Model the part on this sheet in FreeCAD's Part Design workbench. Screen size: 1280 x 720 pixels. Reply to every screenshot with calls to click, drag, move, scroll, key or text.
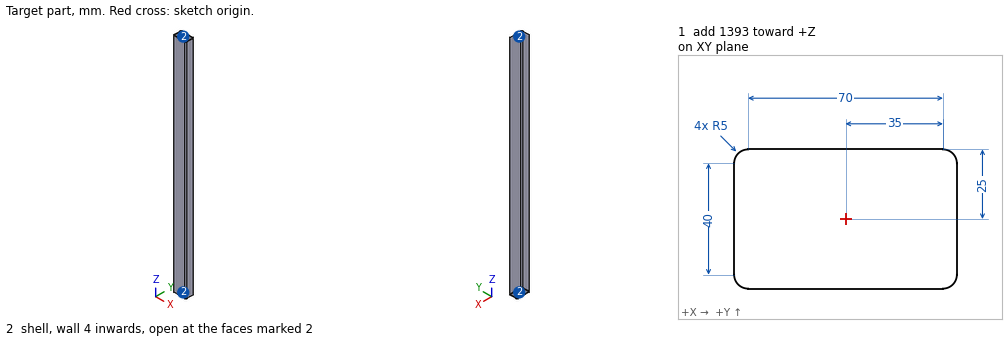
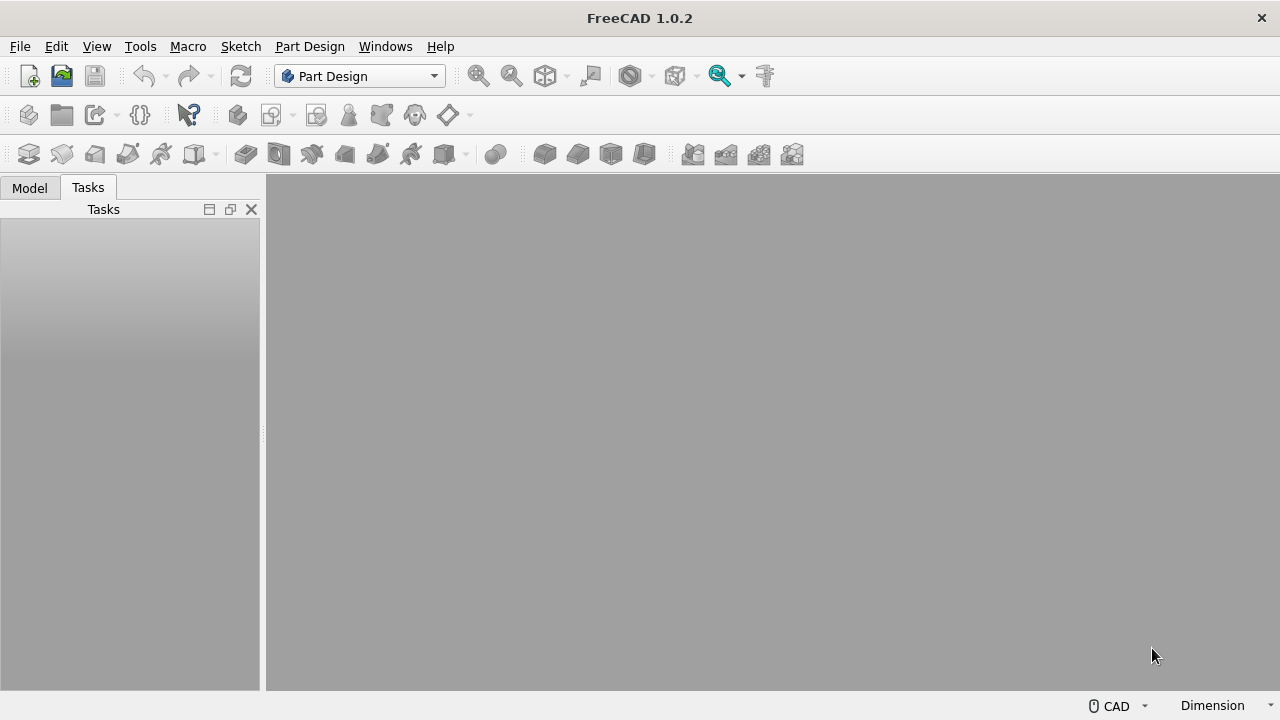
click(29, 76)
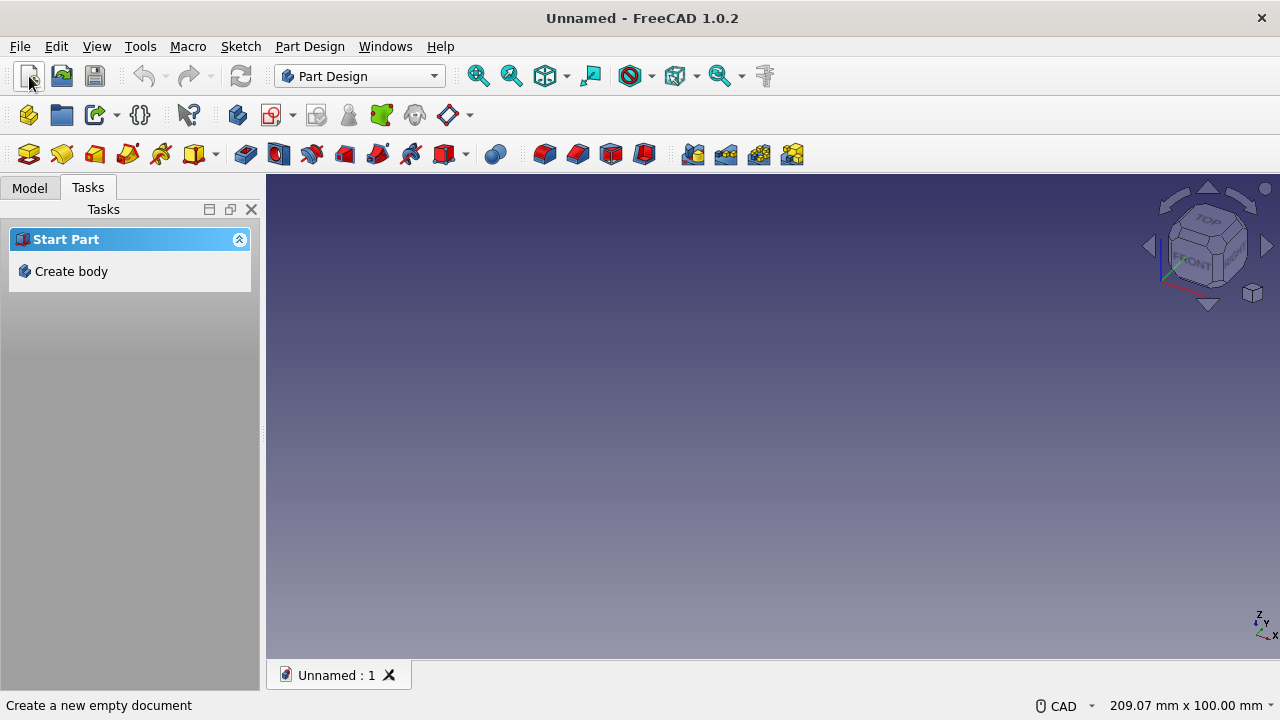
click(270, 116)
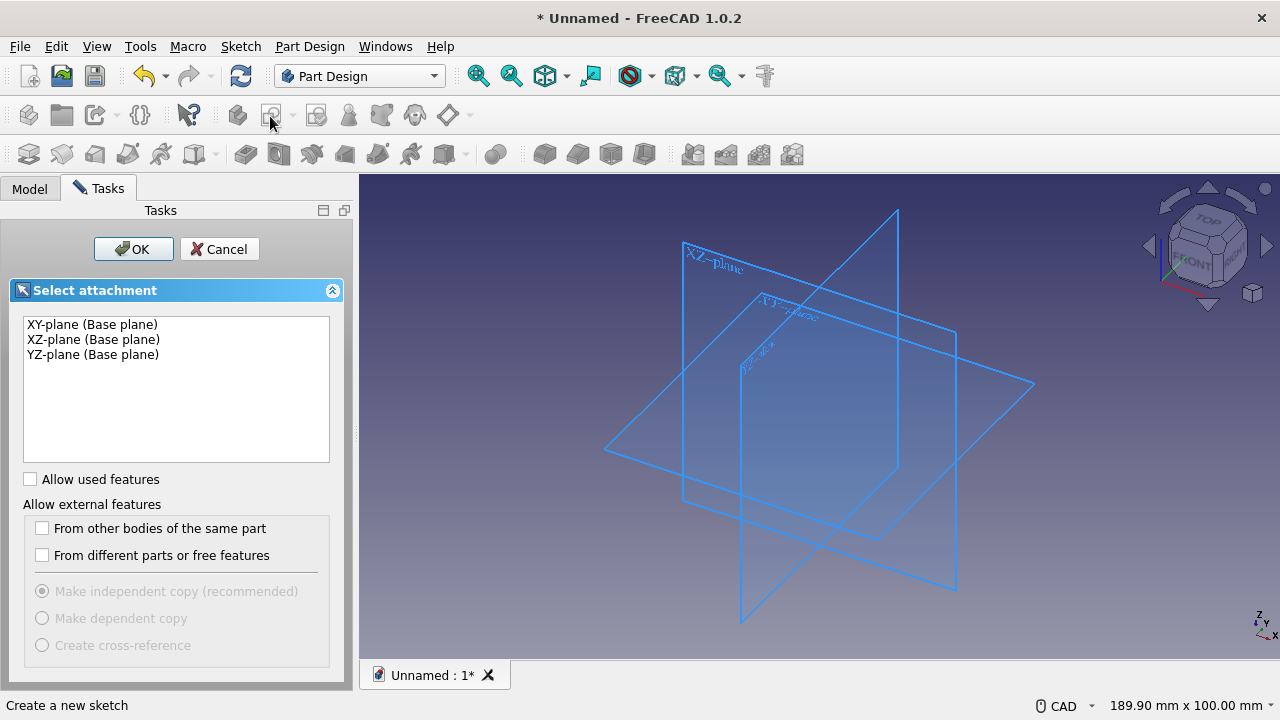
click(84, 324)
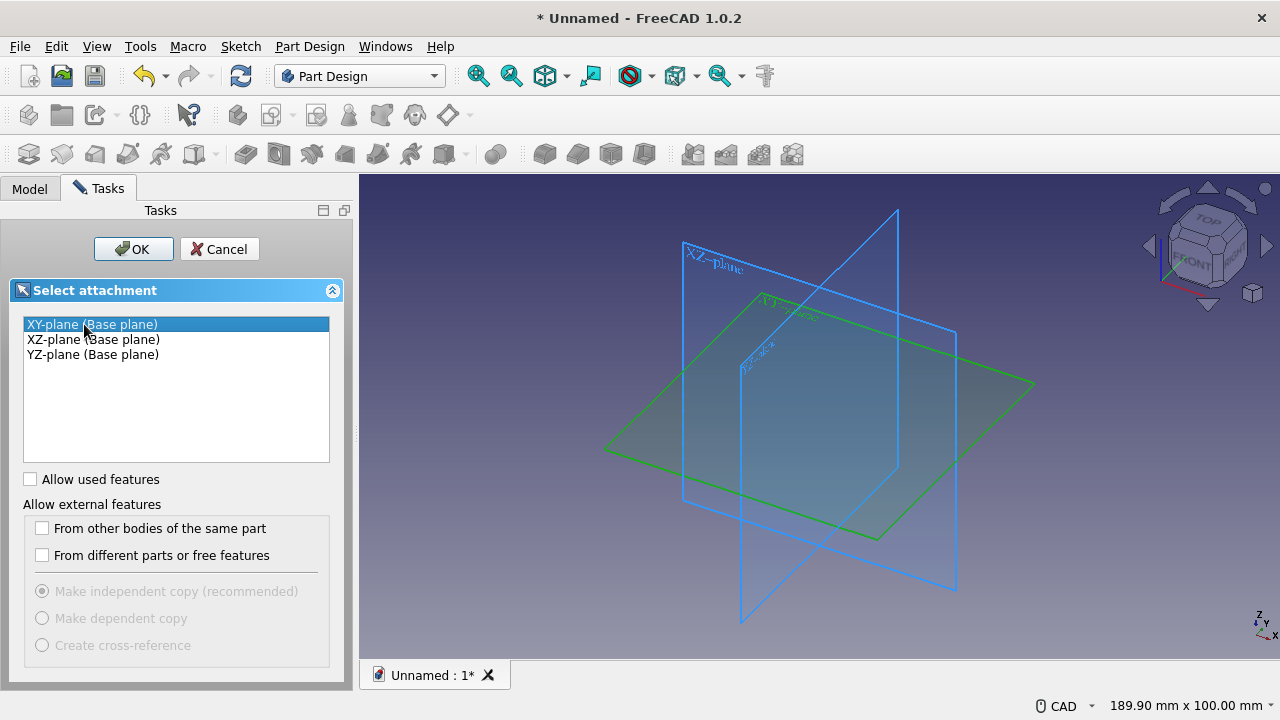
click(134, 249)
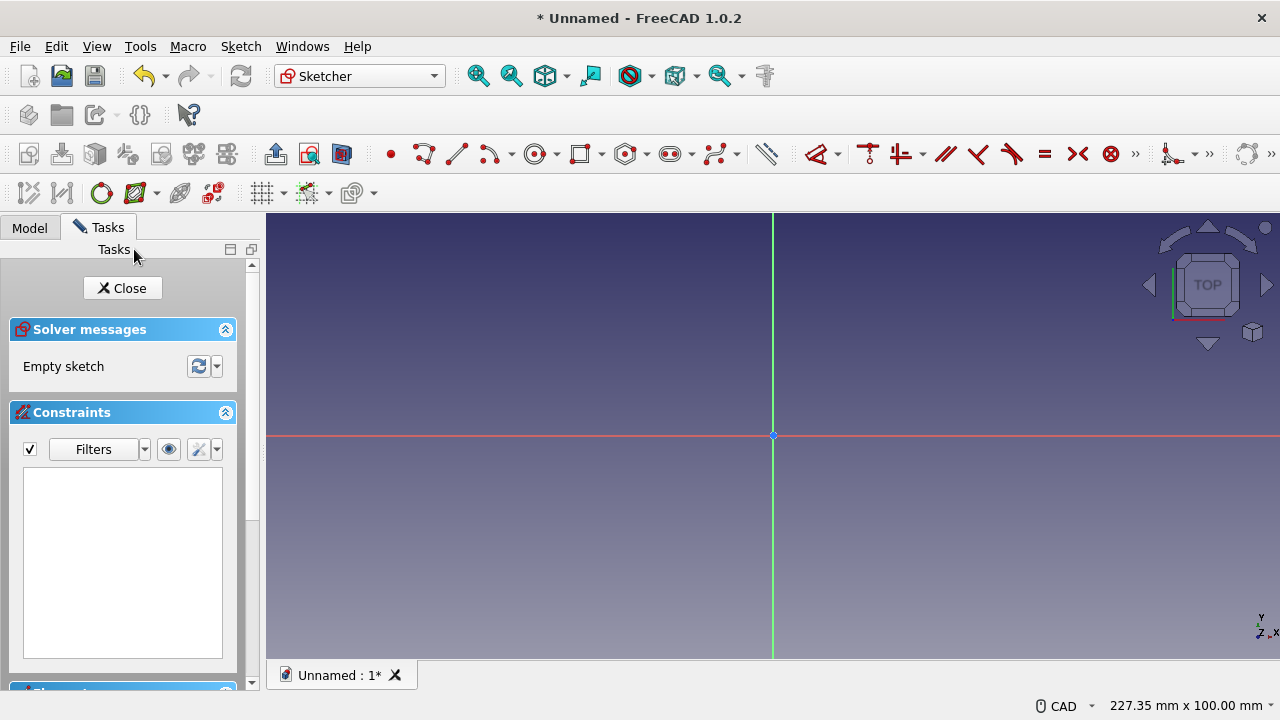
click(457, 154)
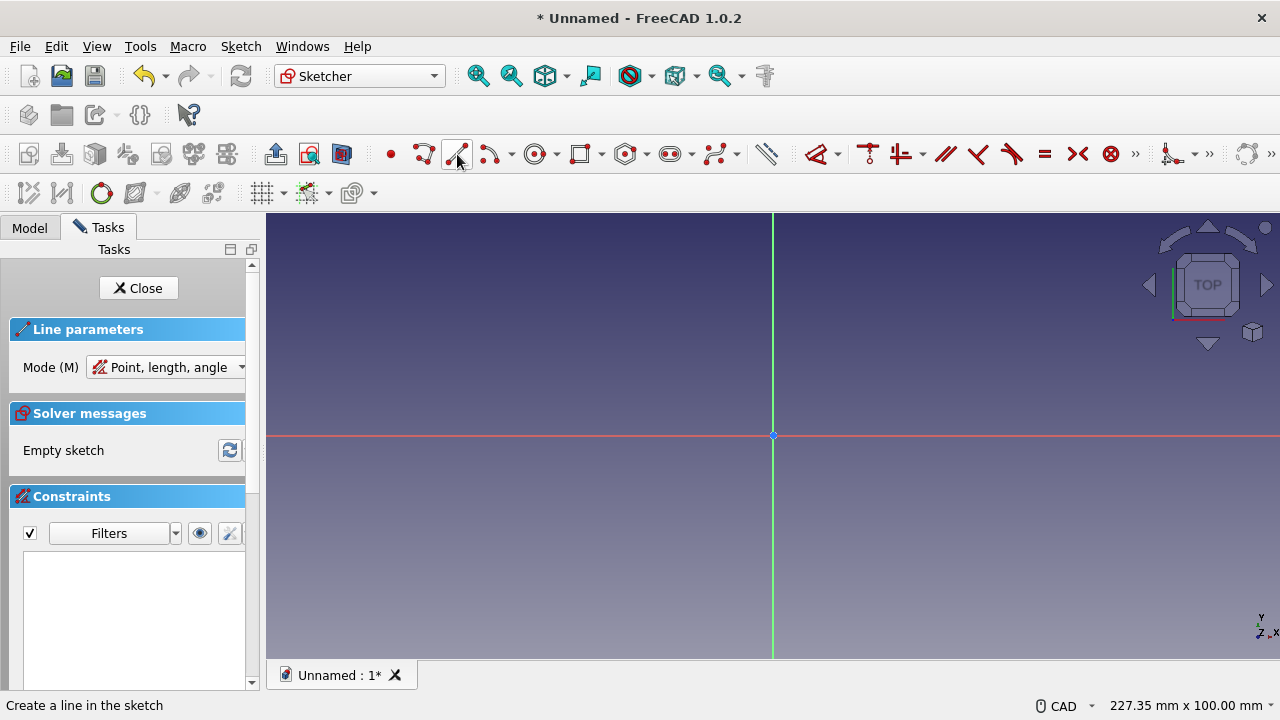
click(929, 324)
click(617, 324)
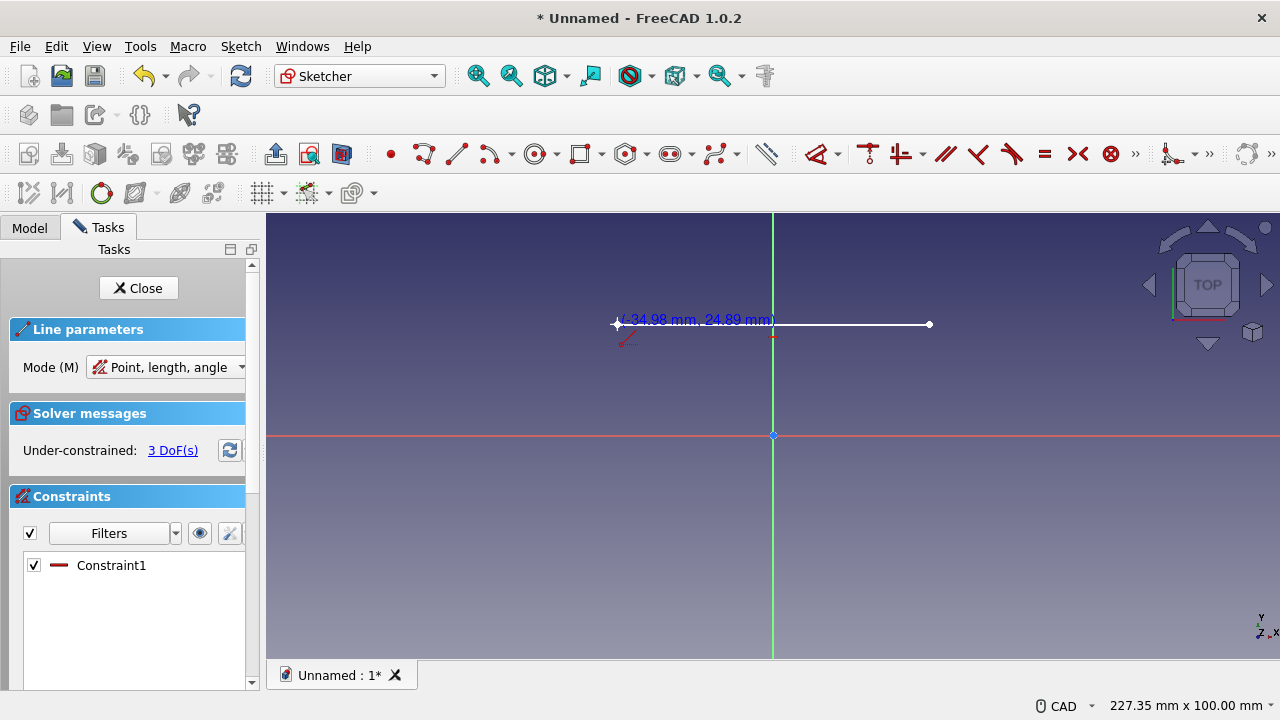
click(595, 347)
click(595, 525)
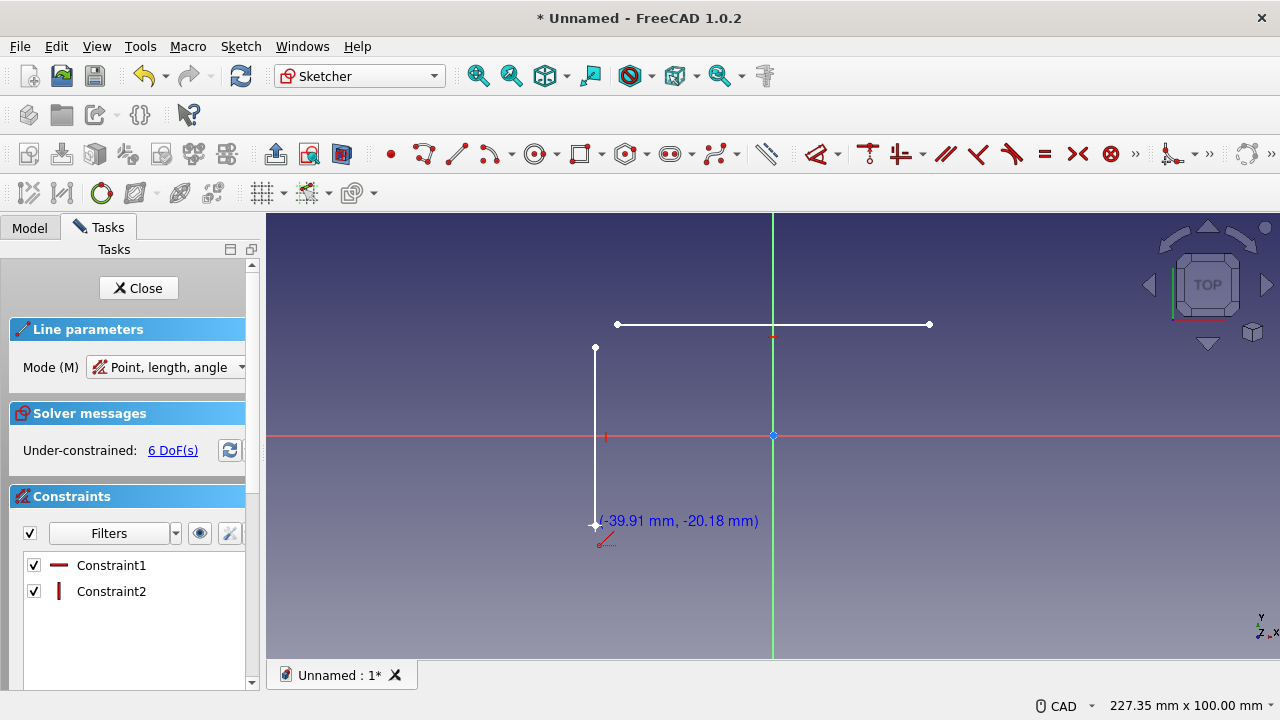
click(617, 548)
click(929, 548)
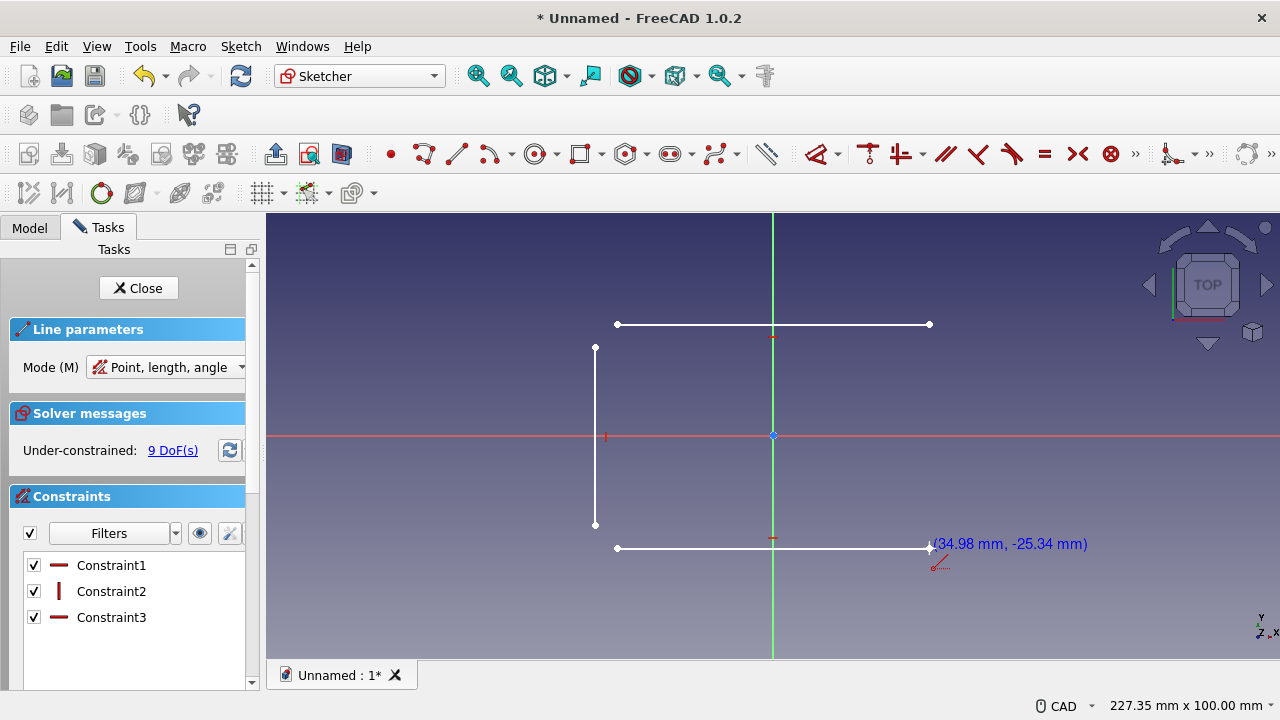
click(951, 525)
click(951, 347)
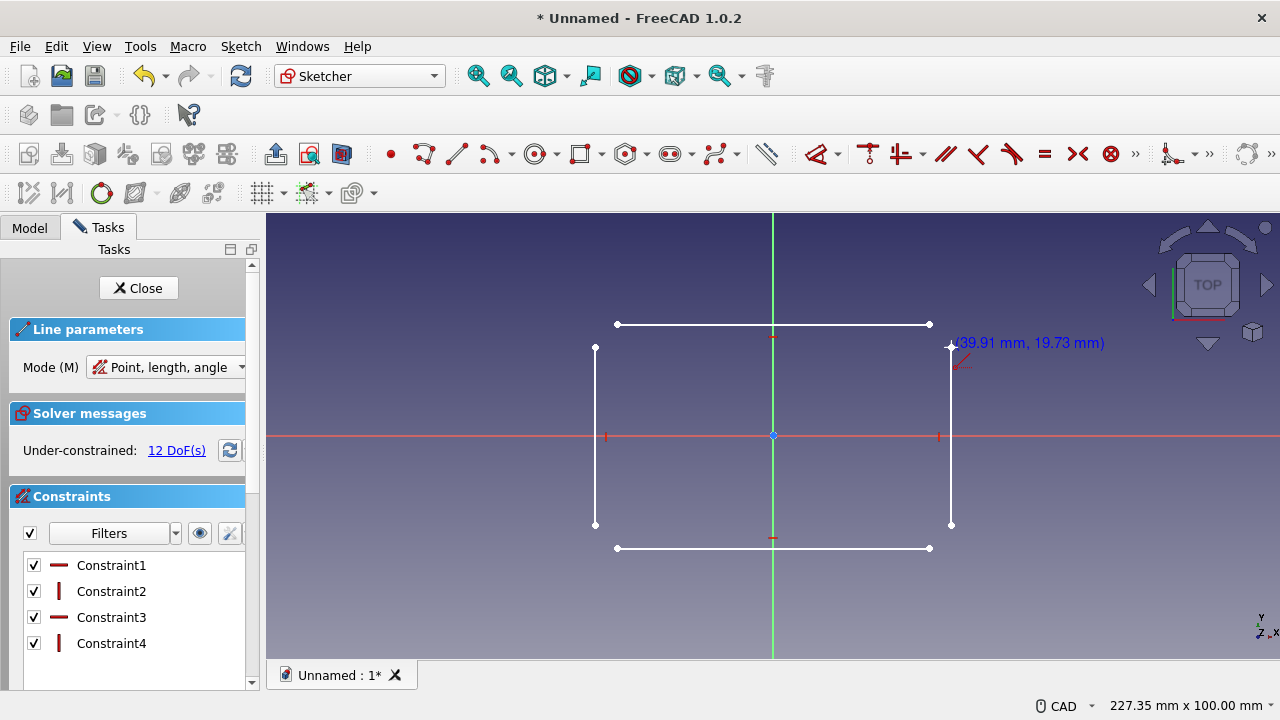
click(512, 154)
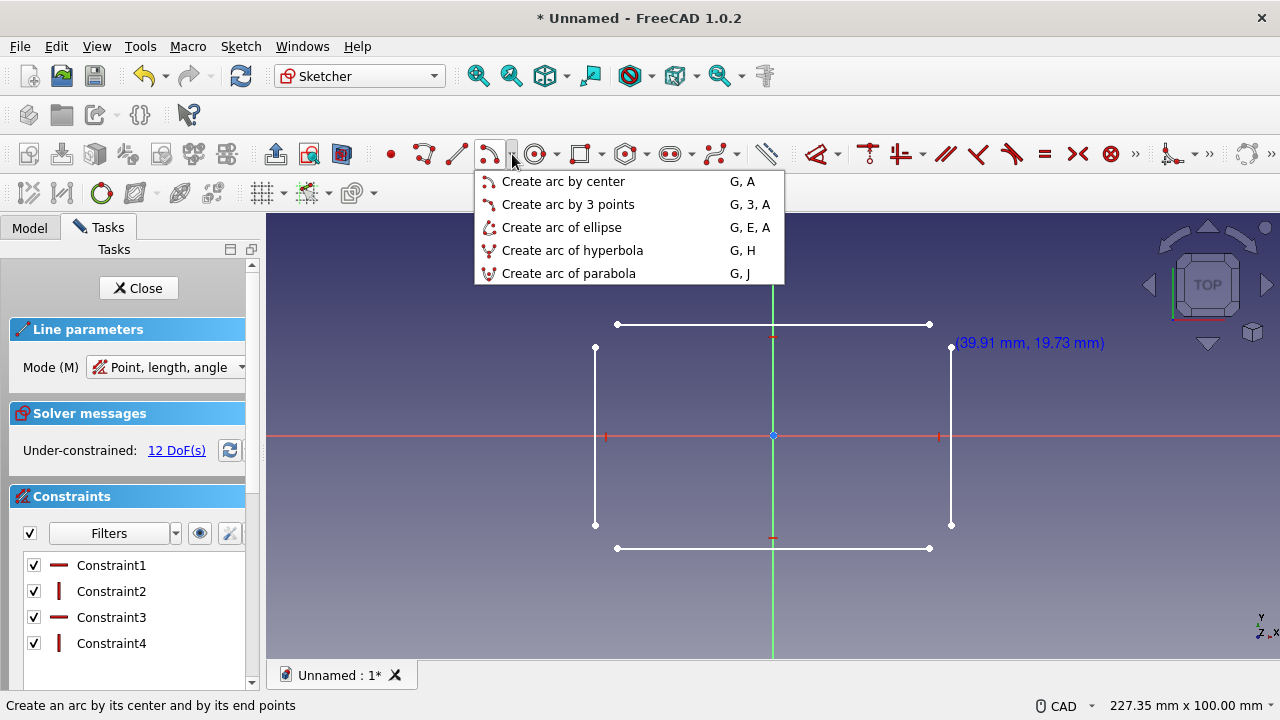
click(630, 204)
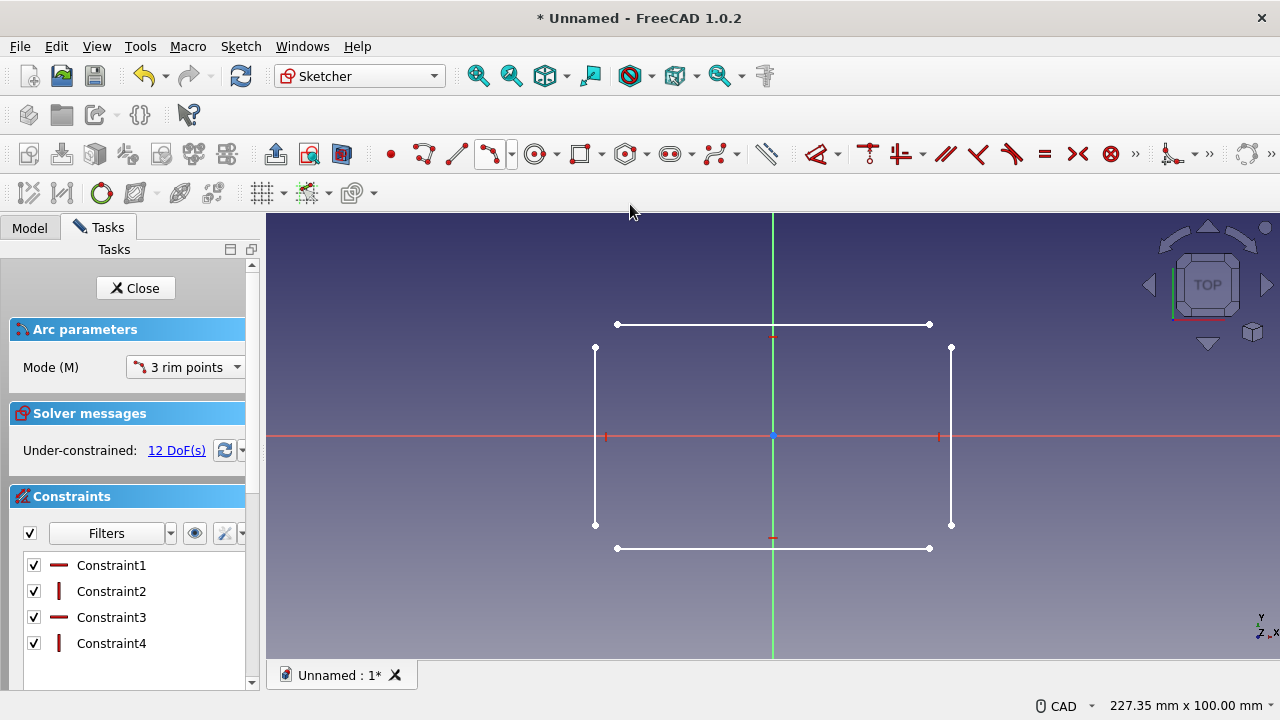
click(617, 325)
click(595, 348)